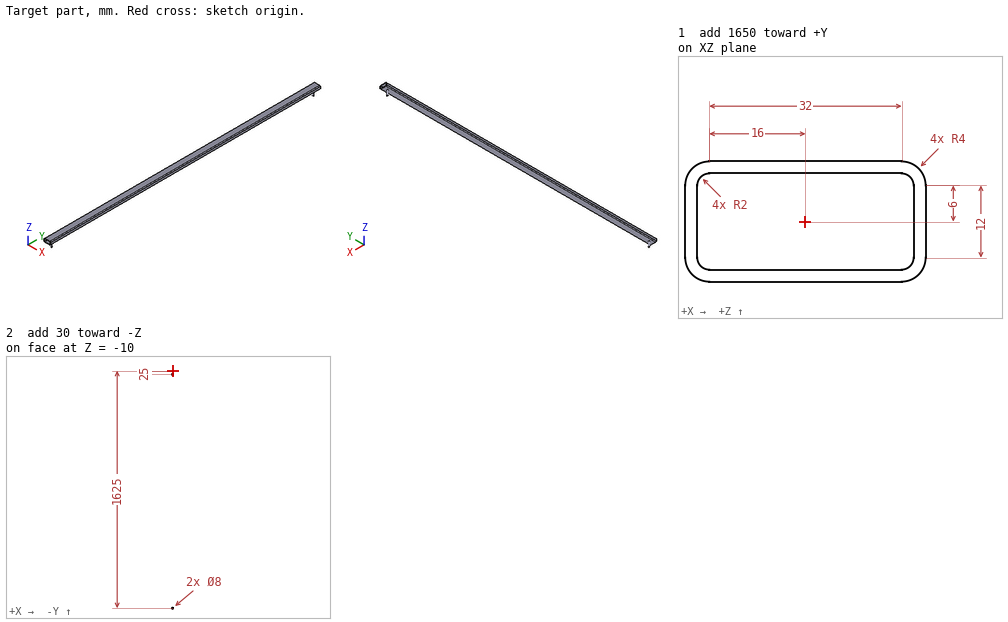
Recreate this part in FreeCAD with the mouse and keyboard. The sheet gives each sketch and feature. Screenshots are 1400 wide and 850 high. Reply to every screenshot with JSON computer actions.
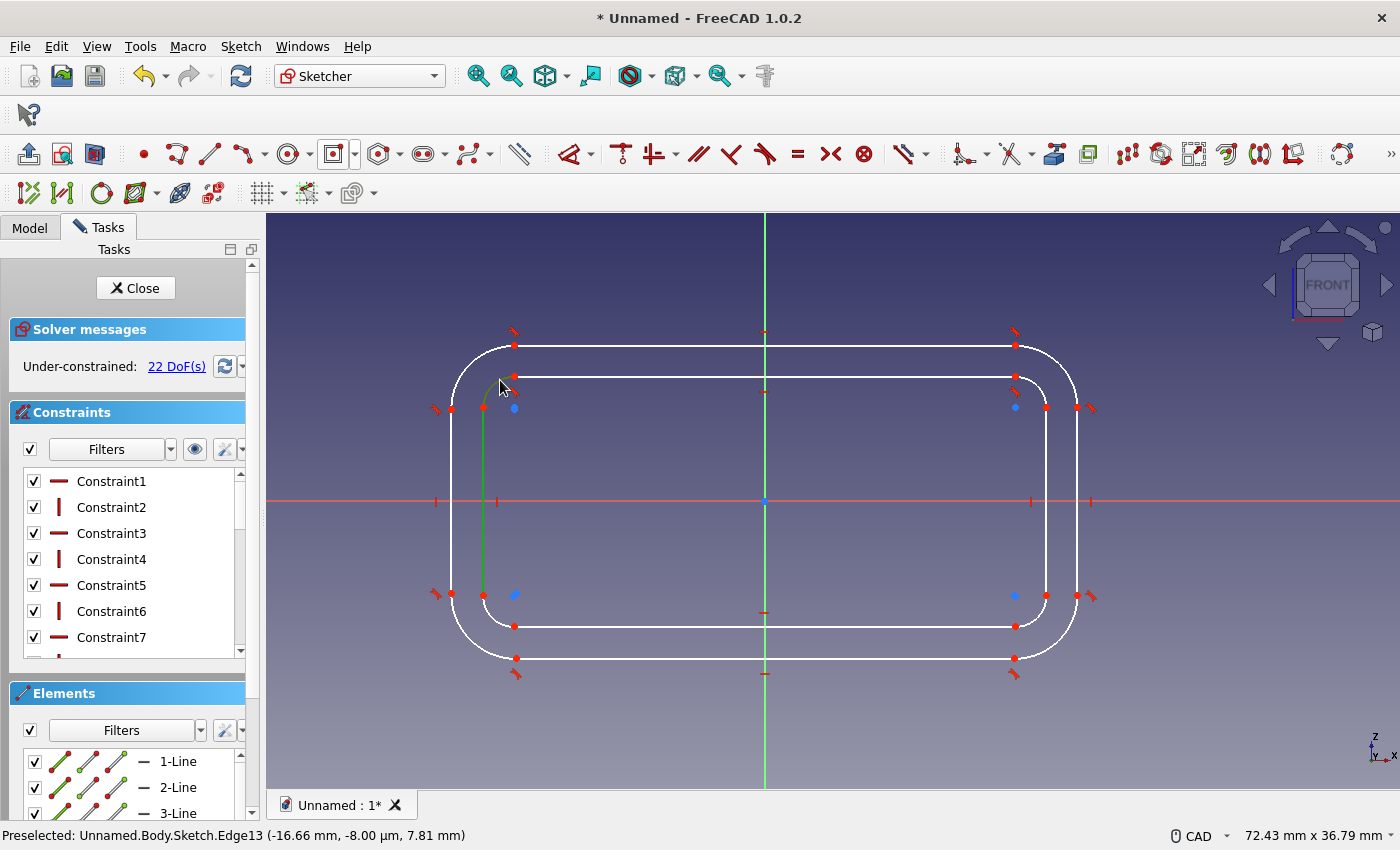
{"action": "left_click", "coordinate": [765, 154]}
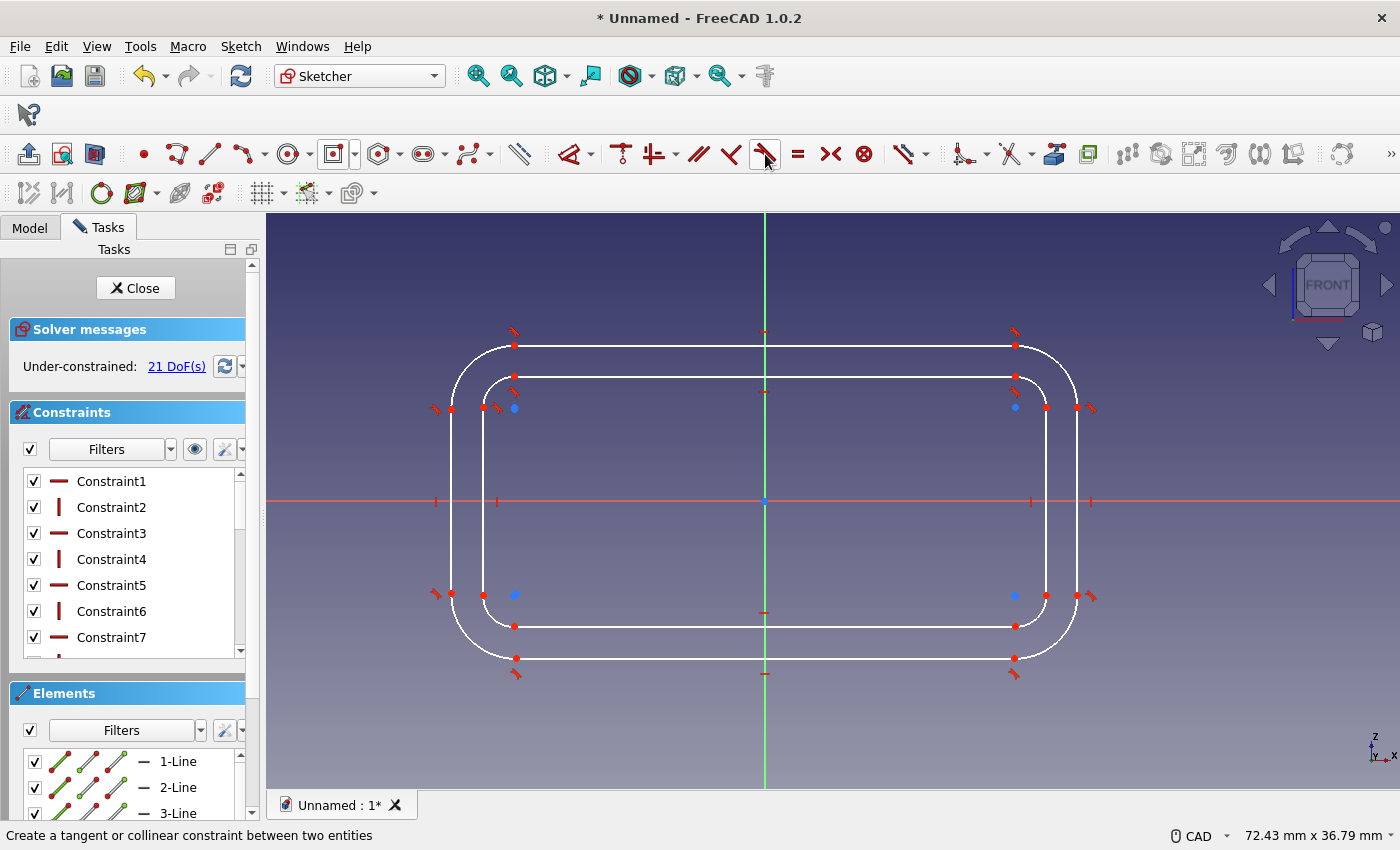
{"action": "left_click", "coordinate": [483, 464]}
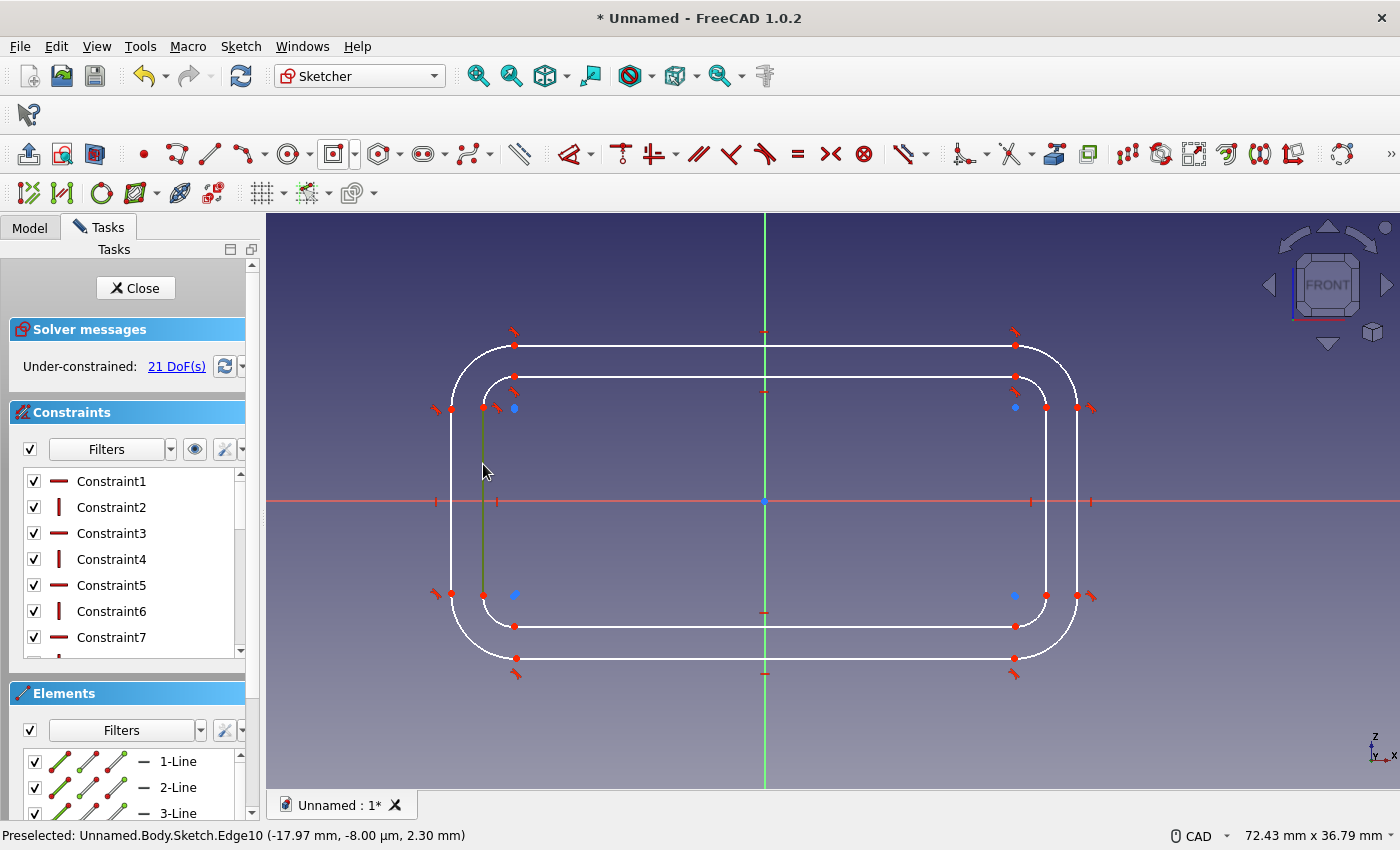
{"action": "left_click", "coordinate": [486, 610]}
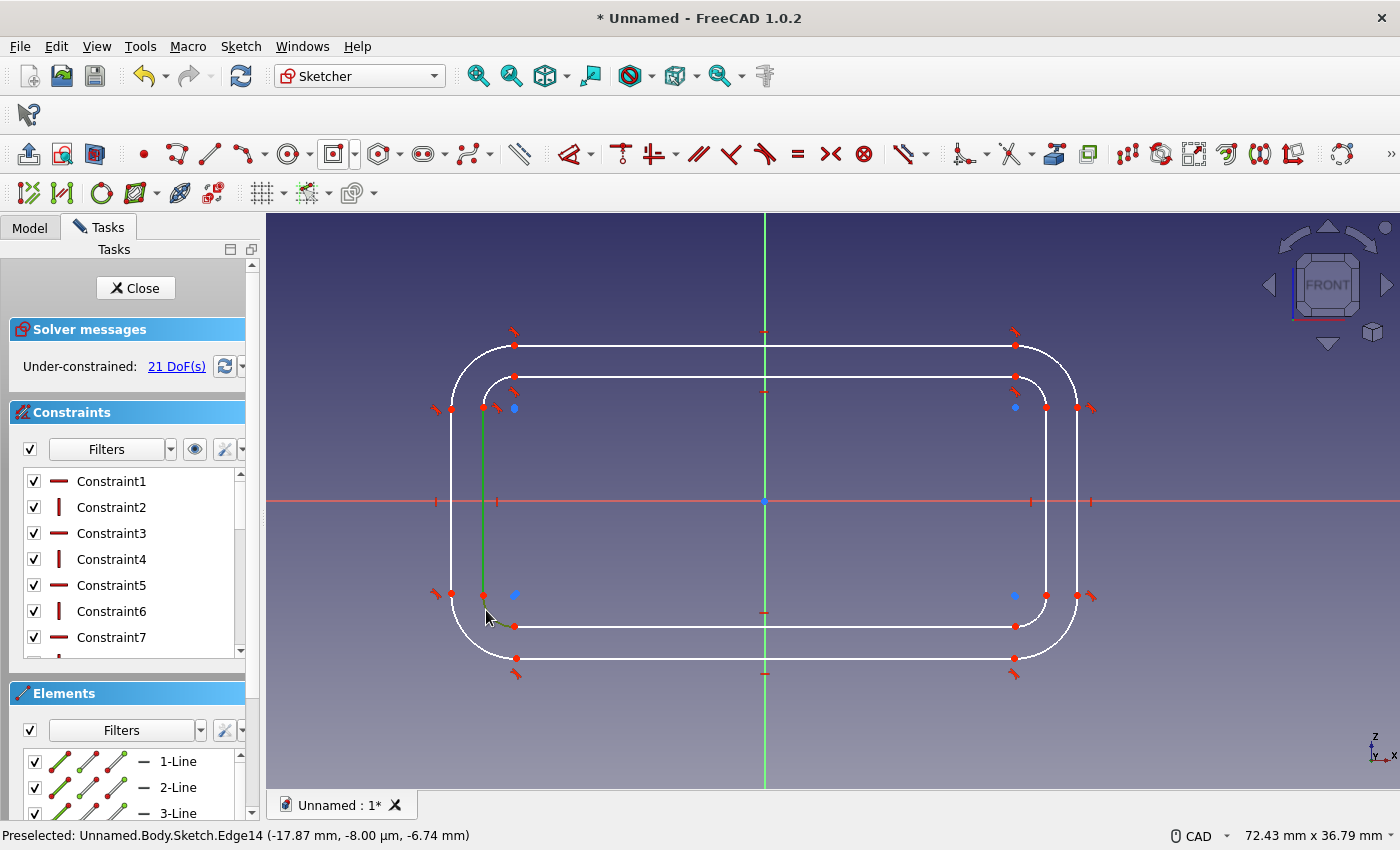
{"action": "left_click", "coordinate": [765, 154]}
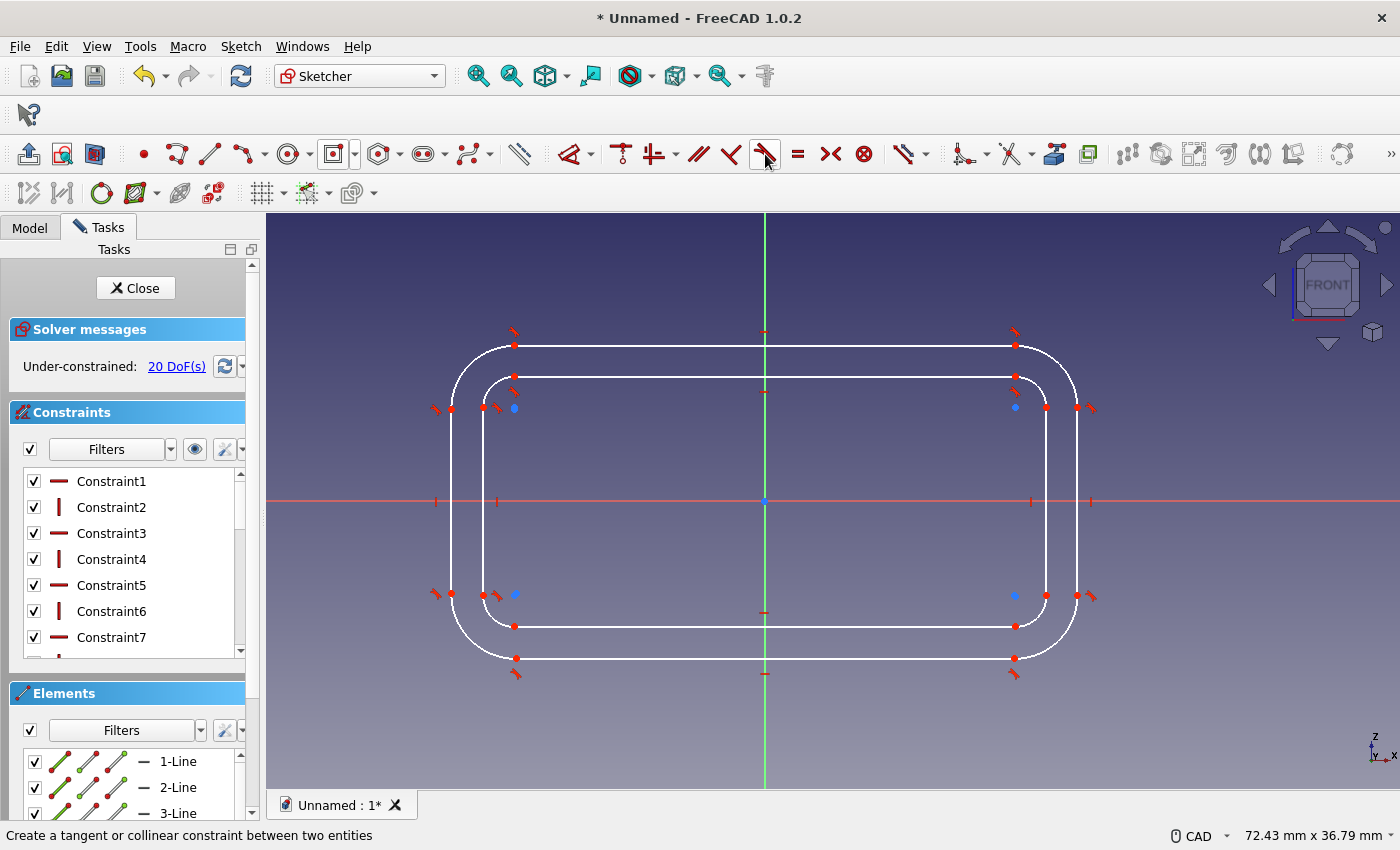
{"action": "left_click", "coordinate": [665, 627]}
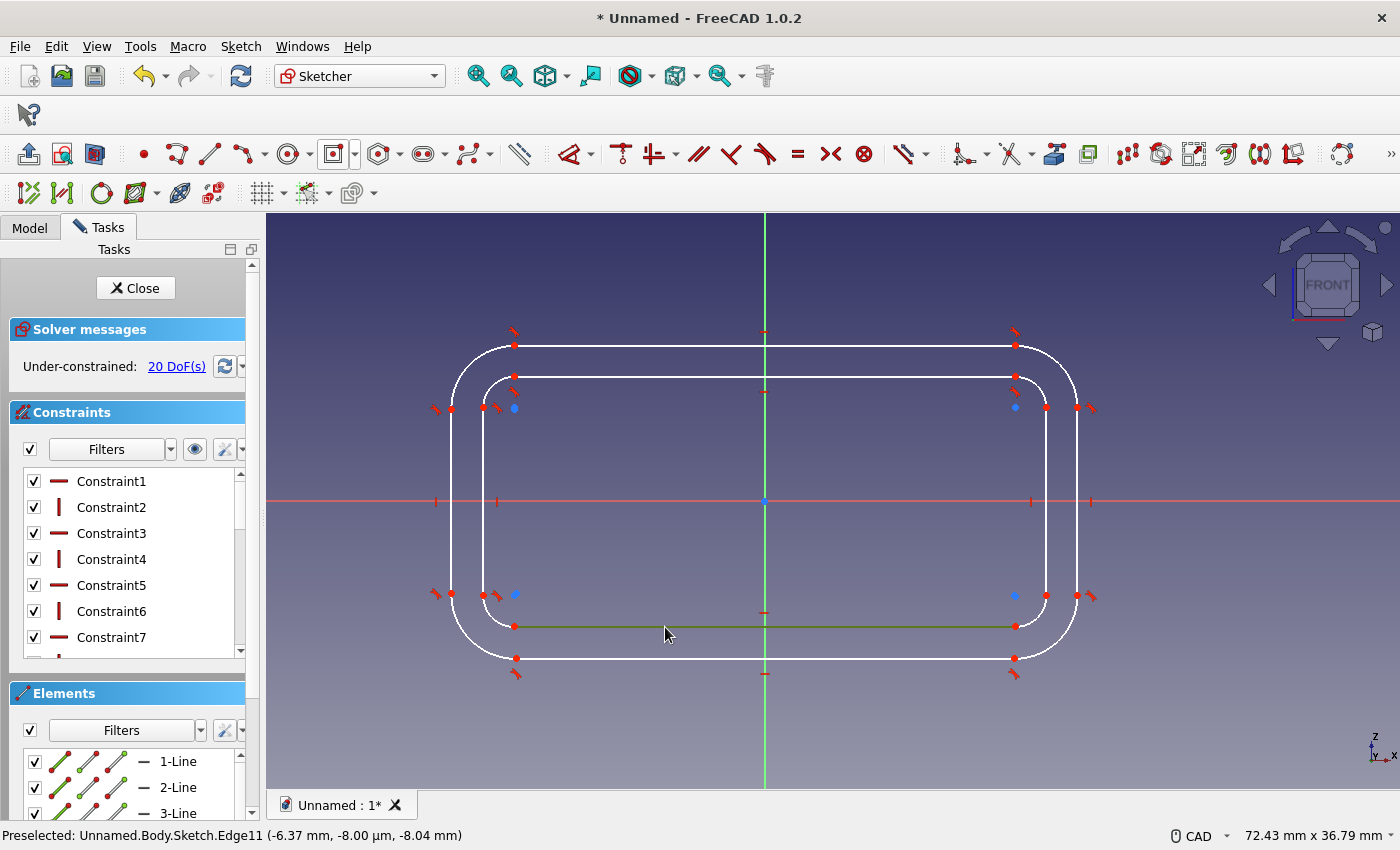
{"action": "left_click", "coordinate": [487, 610]}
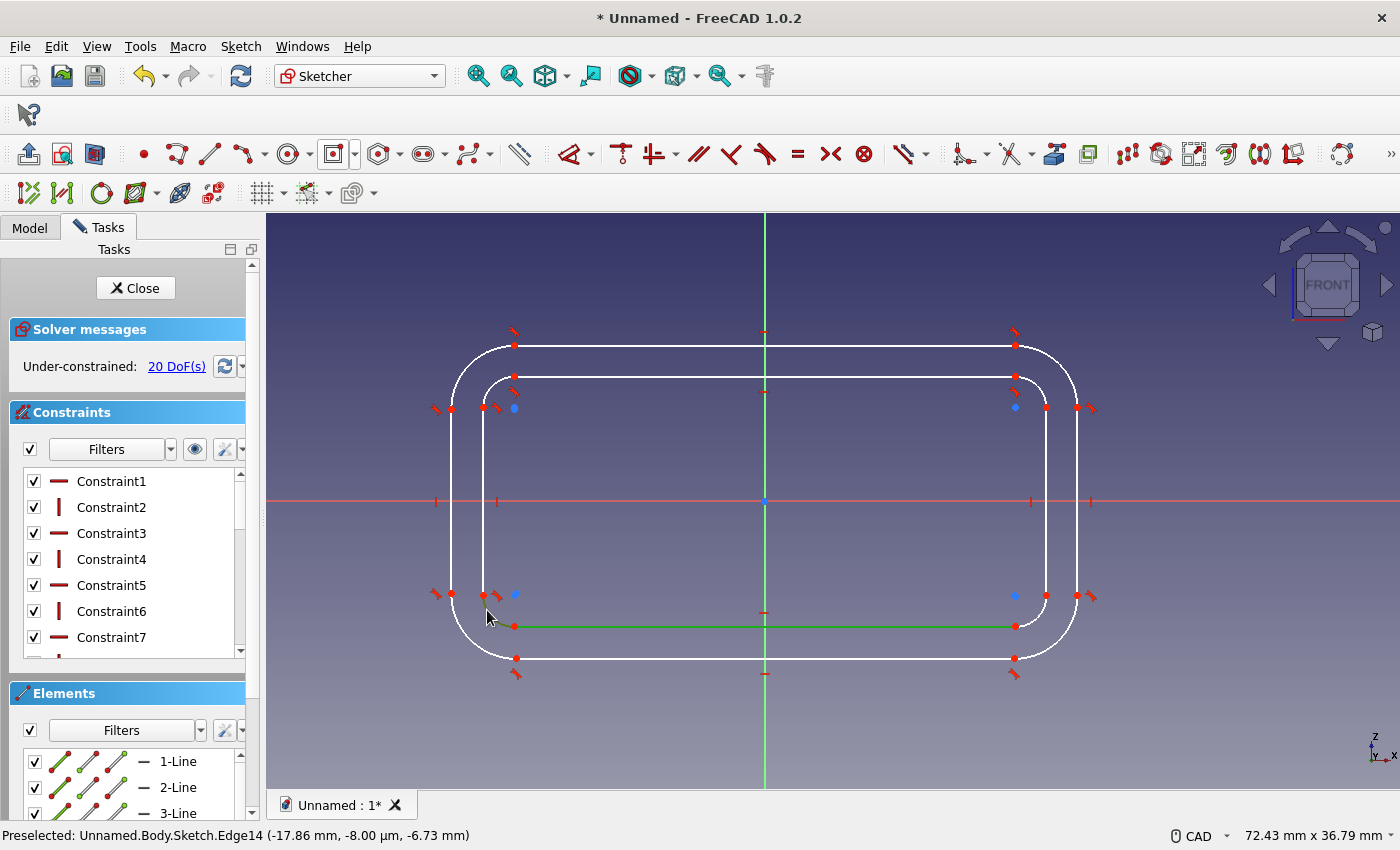
{"action": "left_click", "coordinate": [765, 154]}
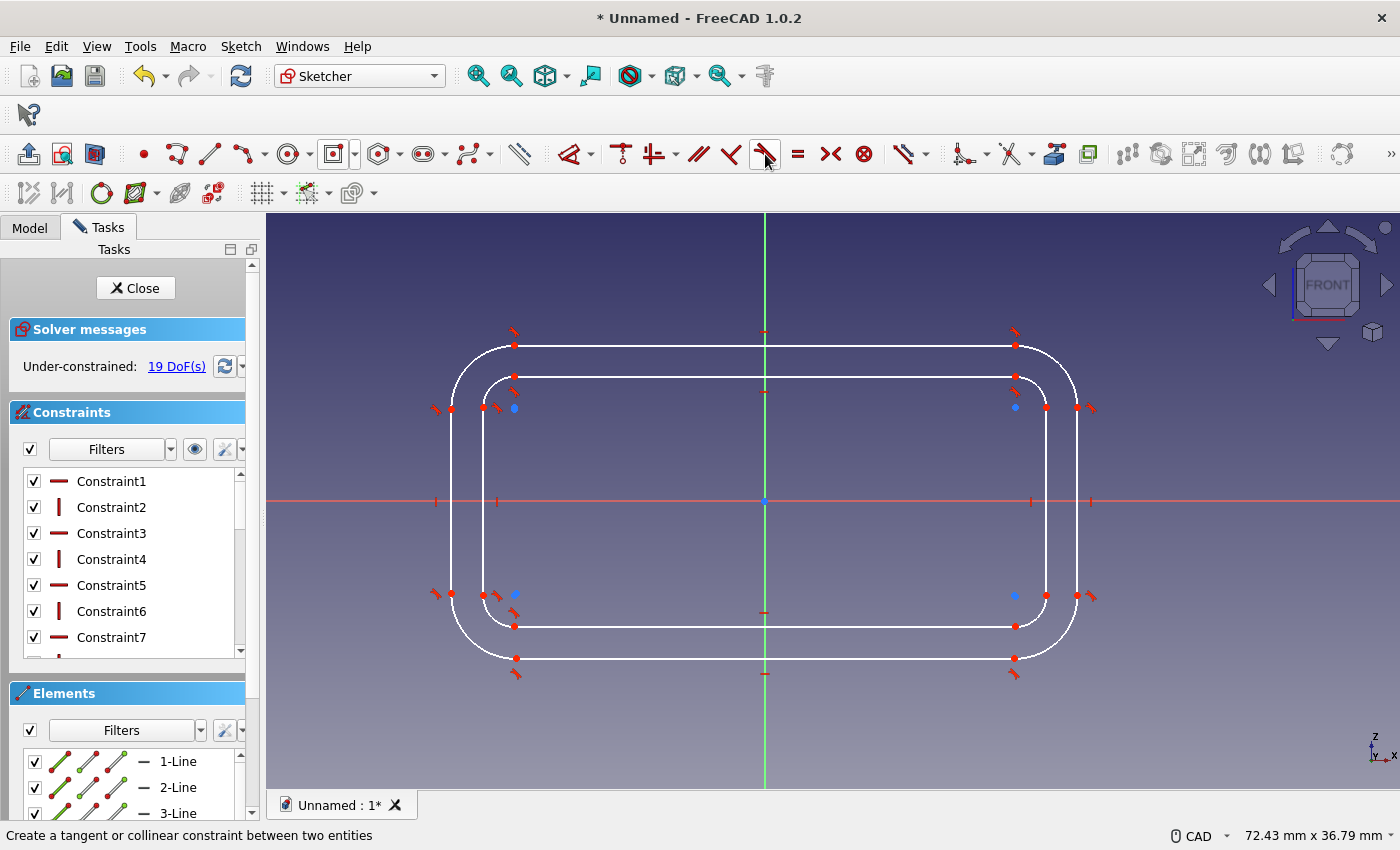
{"action": "left_click", "coordinate": [665, 627]}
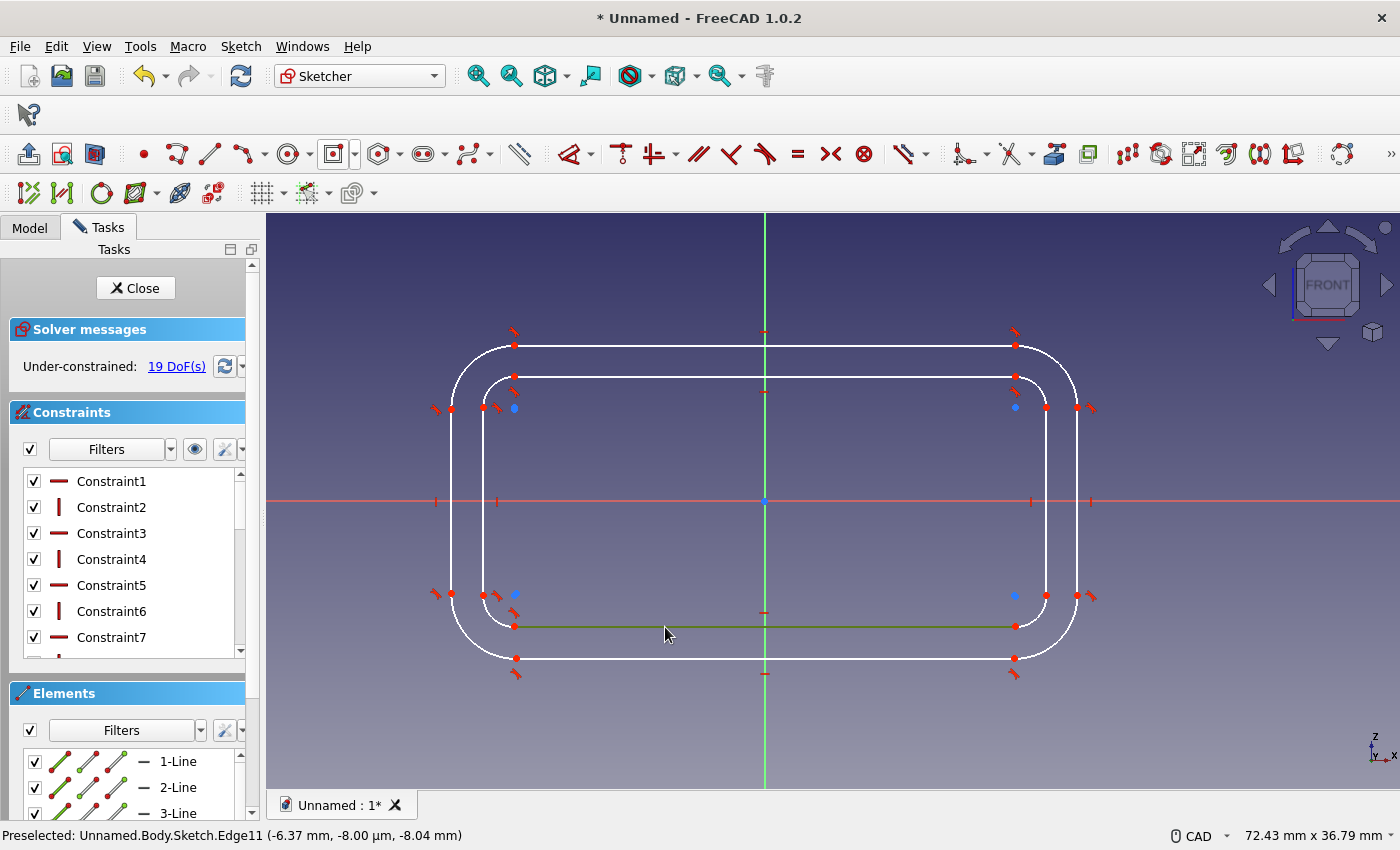
{"action": "left_click", "coordinate": [1029, 624]}